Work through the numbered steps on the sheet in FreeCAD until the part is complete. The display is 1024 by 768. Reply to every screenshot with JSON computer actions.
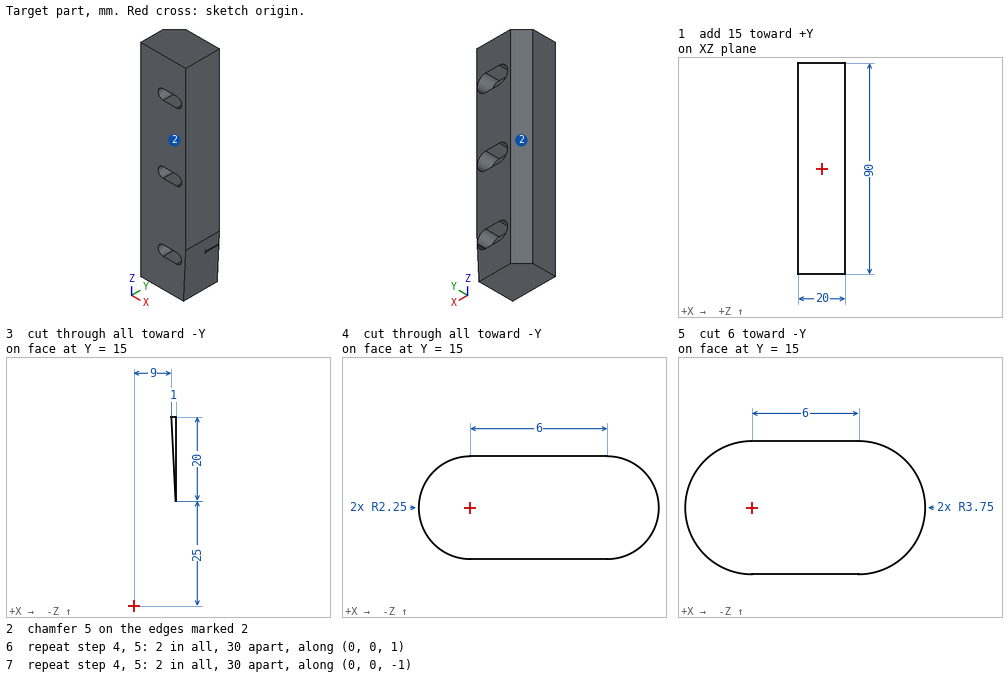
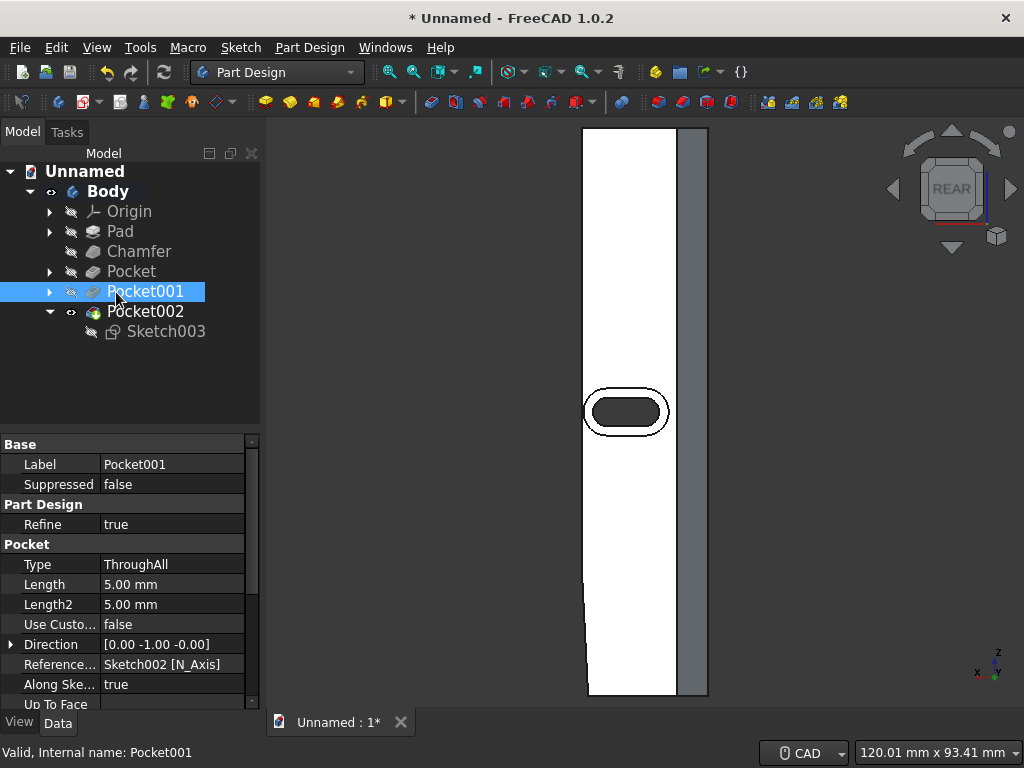
{"action": "left_click", "coordinate": [116, 312], "text": "ctrl"}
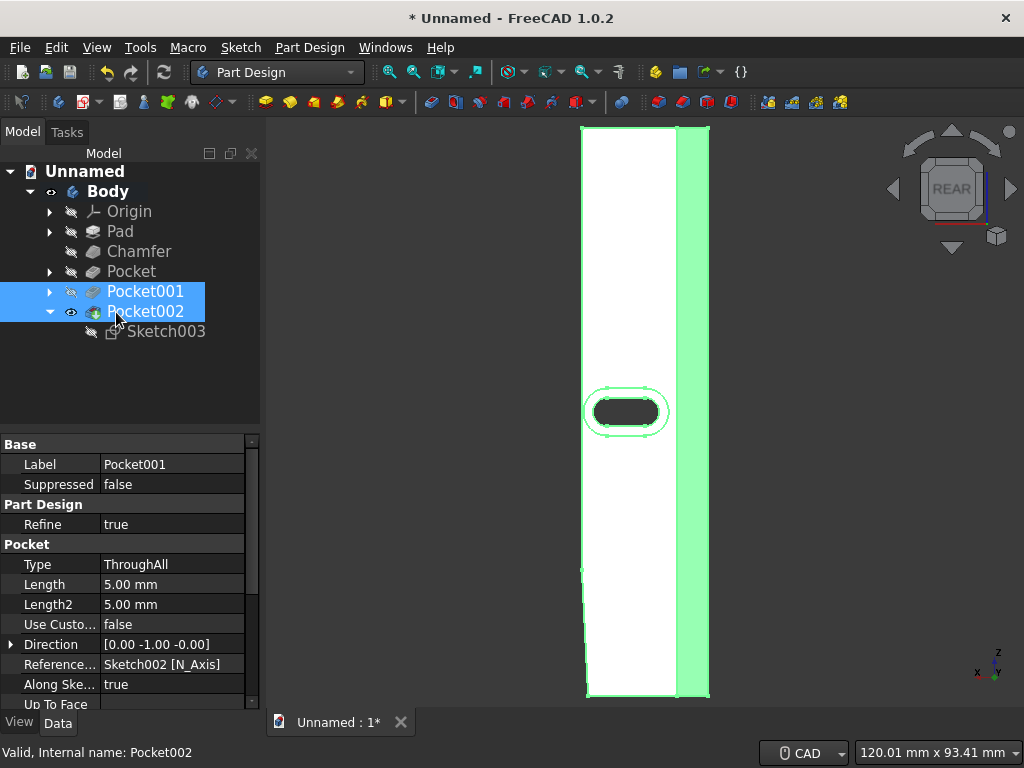
{"action": "left_click", "coordinate": [792, 102]}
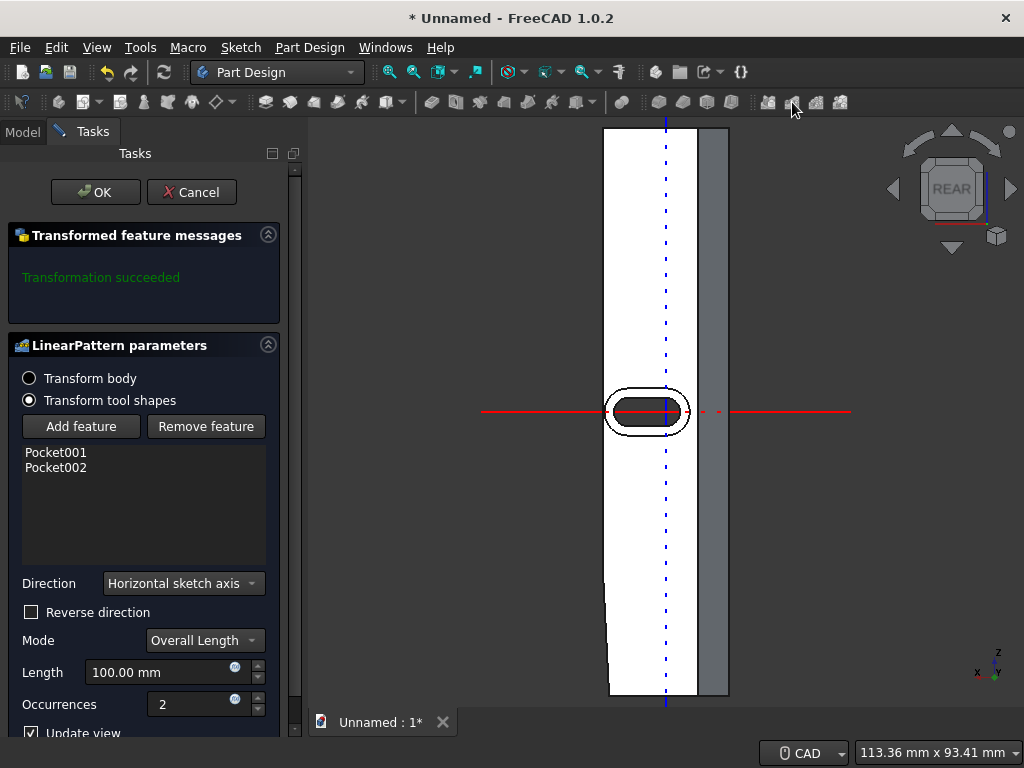
{"action": "left_click", "coordinate": [184, 584]}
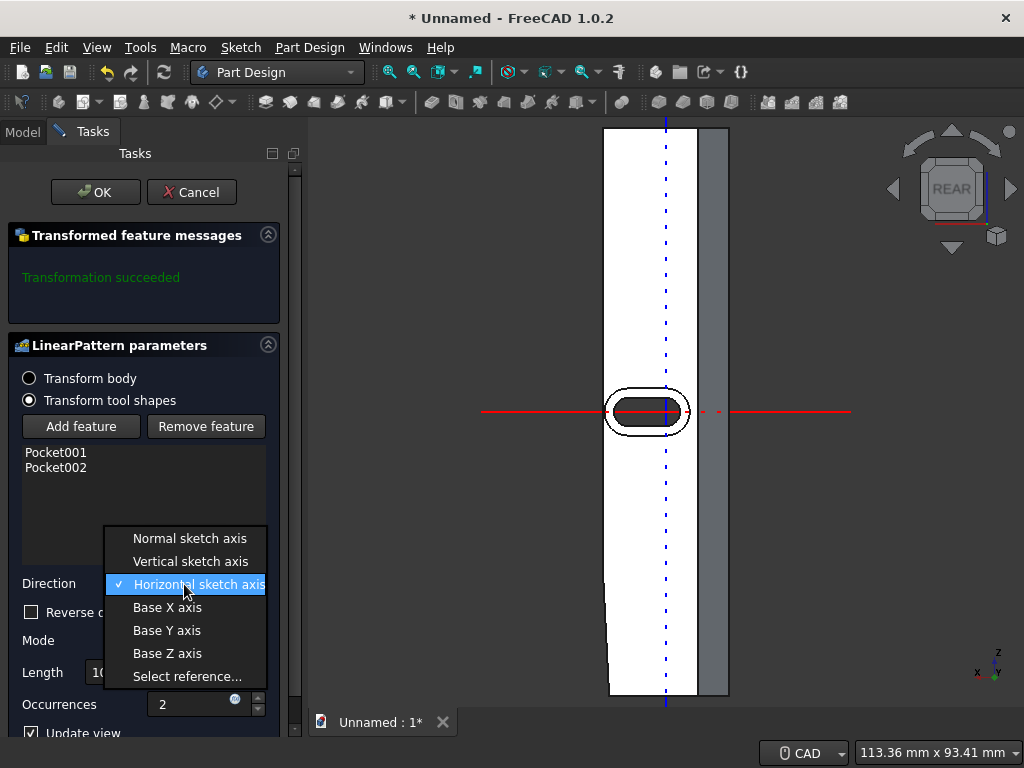
{"action": "left_click", "coordinate": [184, 654]}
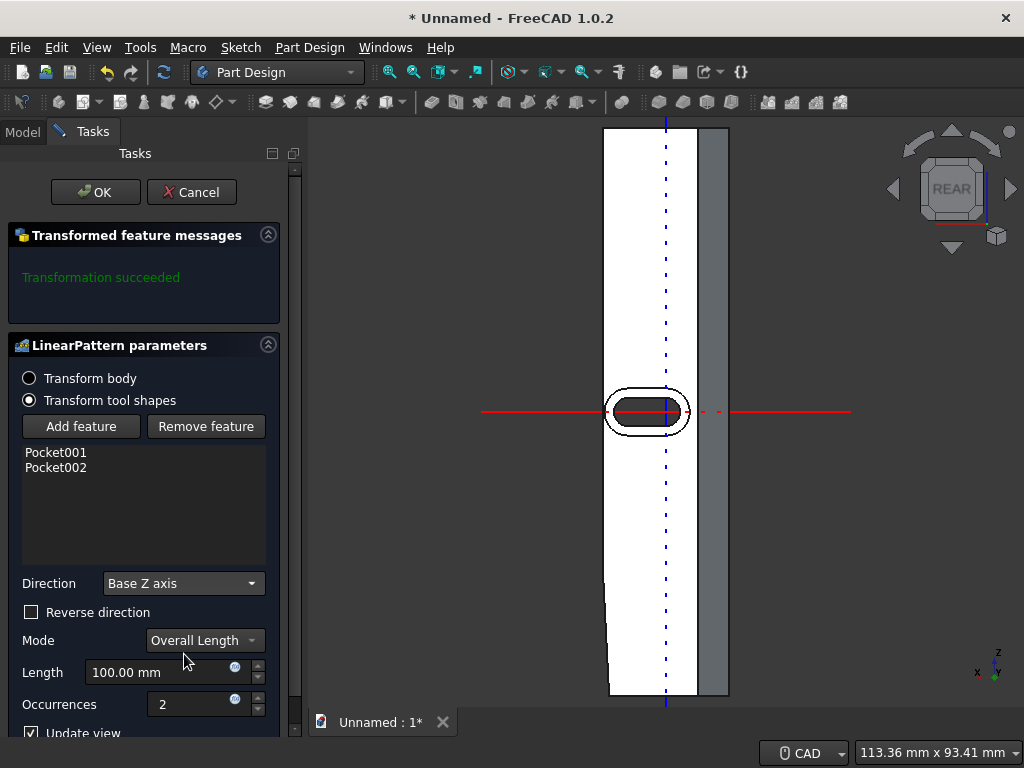
{"action": "left_click", "coordinate": [206, 640]}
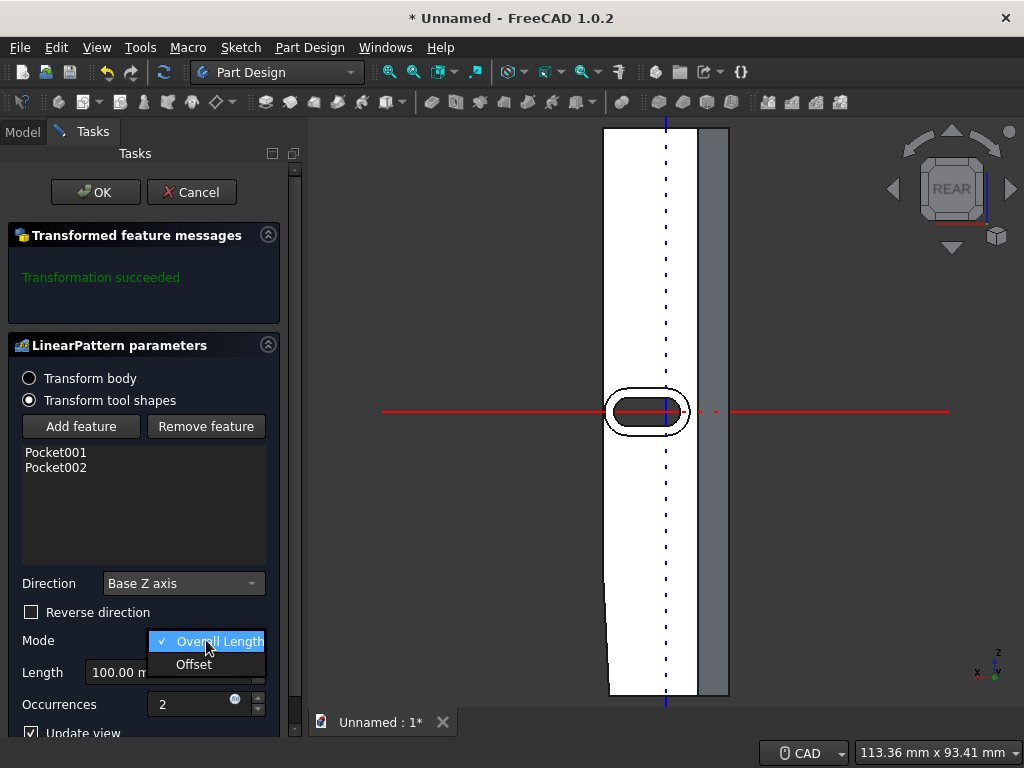
{"action": "left_click", "coordinate": [206, 664]}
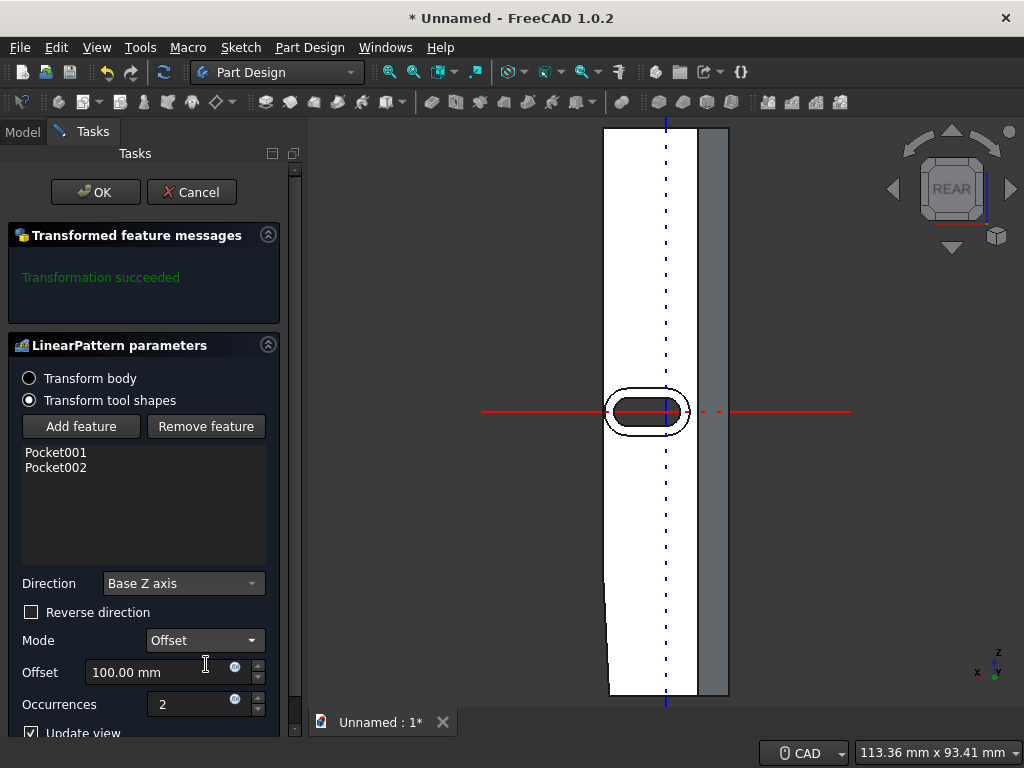
{"action": "triple_click", "coordinate": [168, 672]}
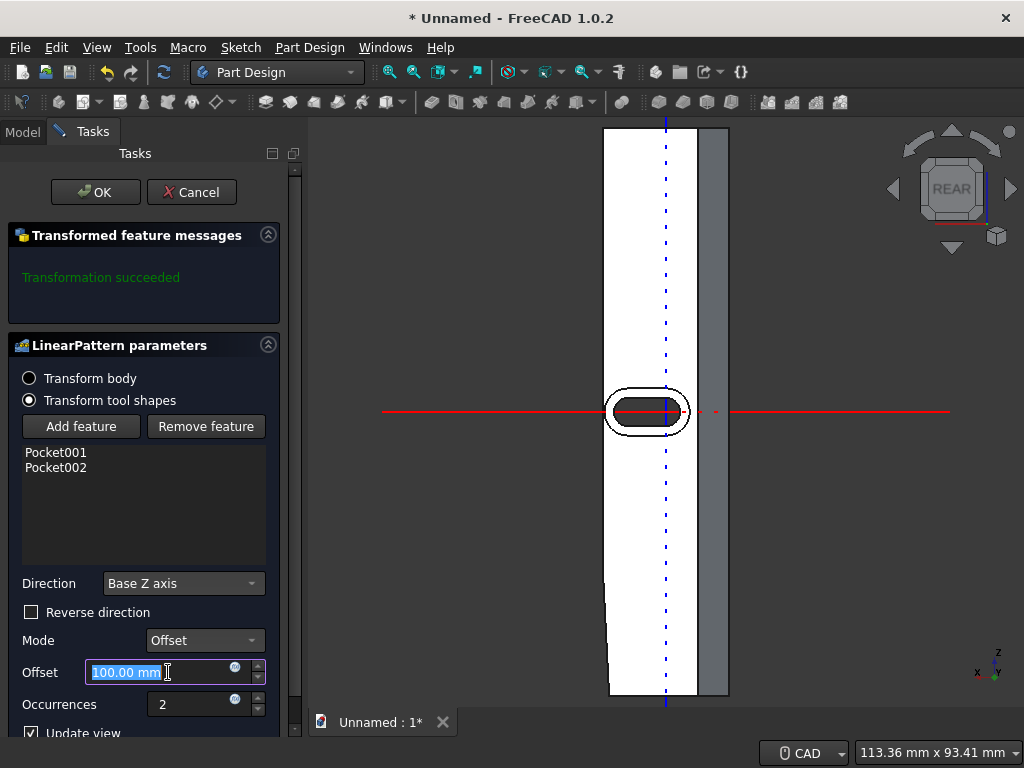
{"action": "type", "text": "30"}
{"action": "key", "text": "Tab"}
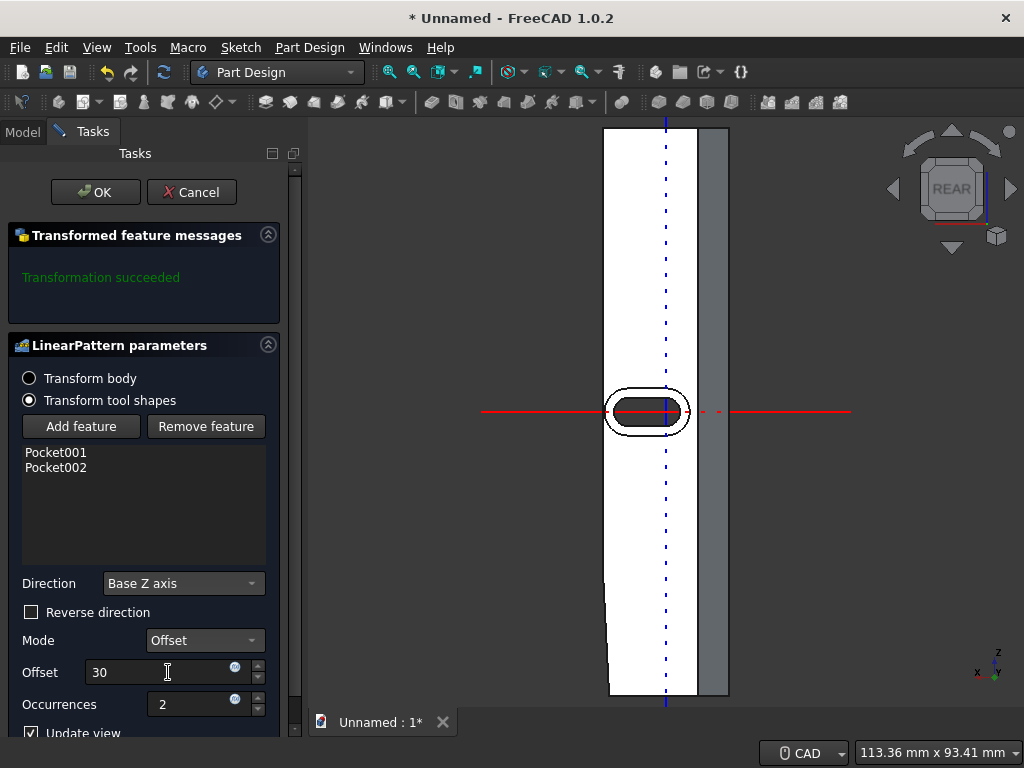
{"action": "triple_click", "coordinate": [198, 704]}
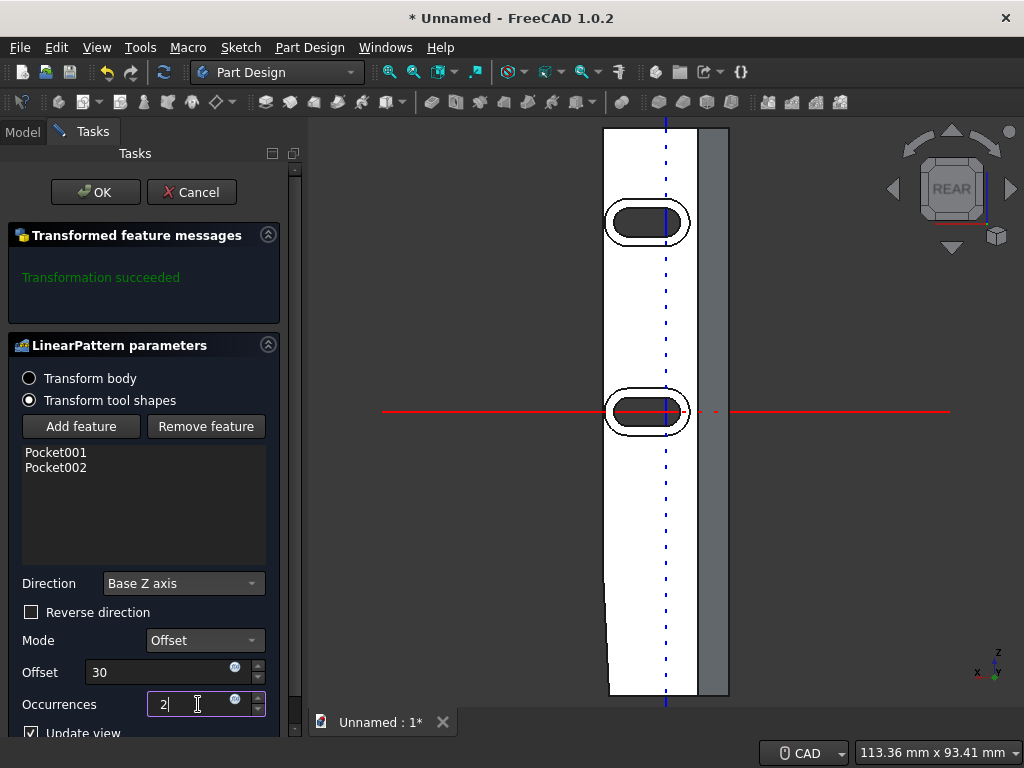
{"action": "type", "text": "2"}
{"action": "key", "text": "Tab"}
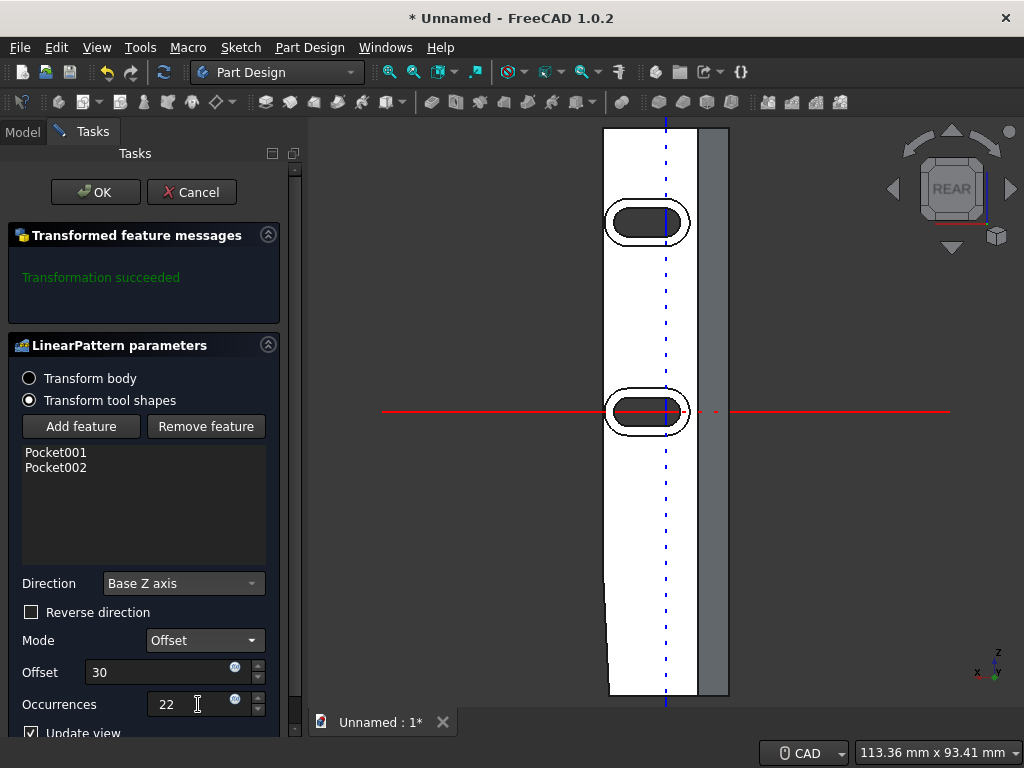
{"action": "left_click", "coordinate": [96, 192]}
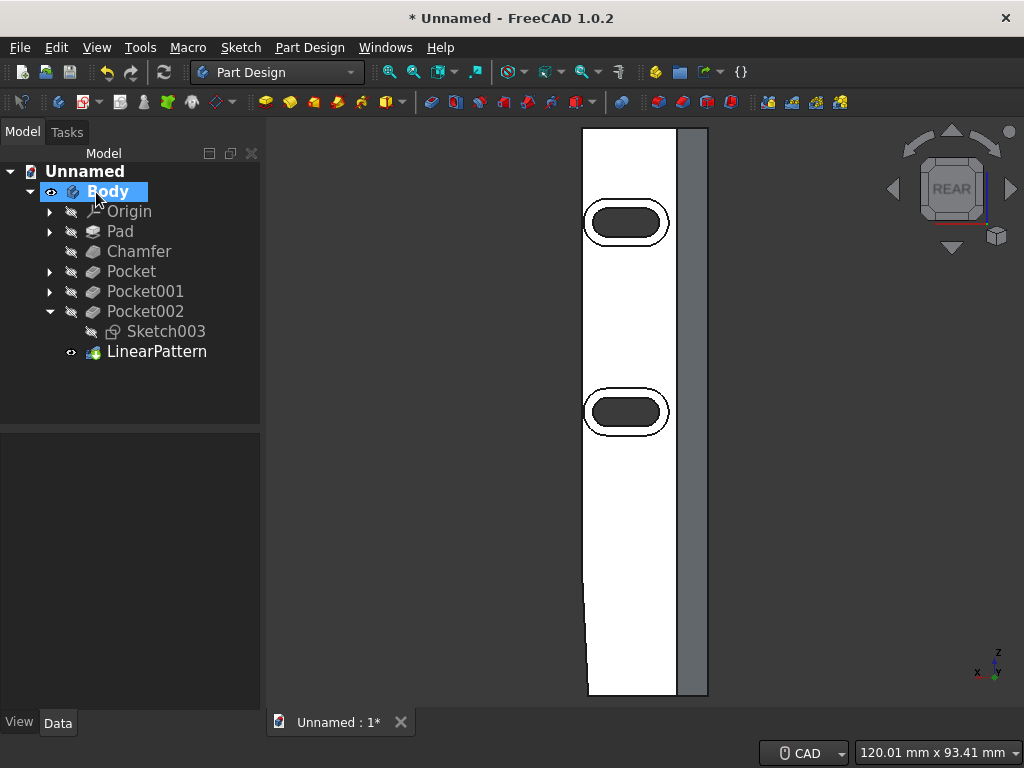
{"action": "left_click", "coordinate": [116, 292]}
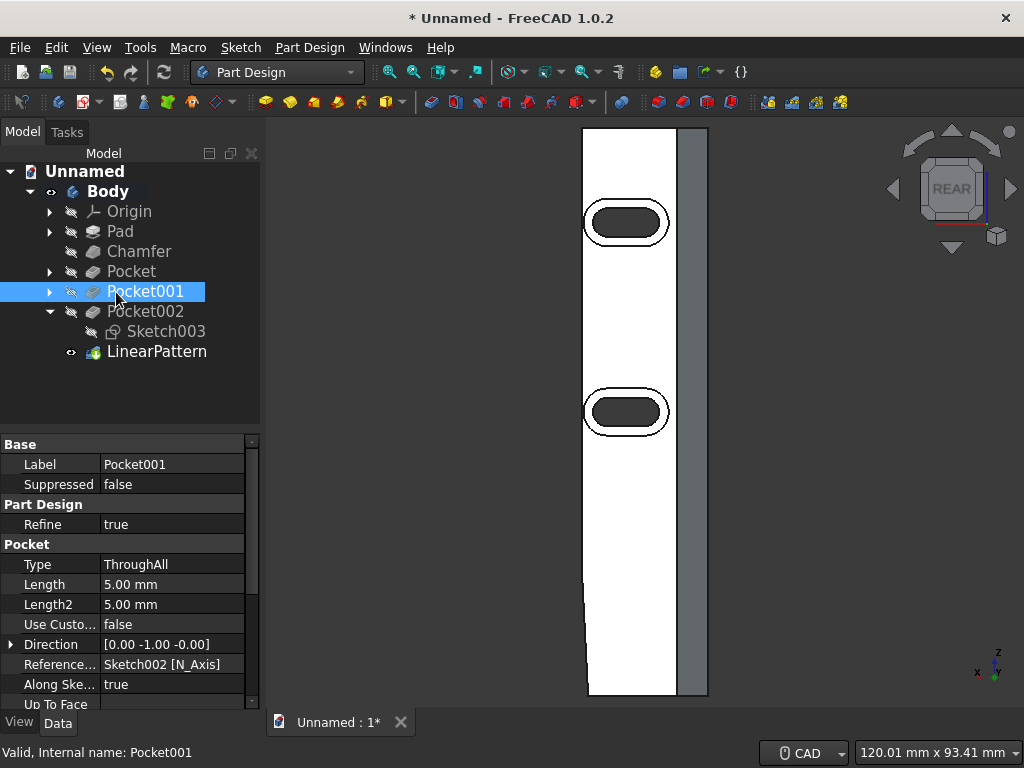
{"action": "left_click", "coordinate": [116, 312], "text": "ctrl"}